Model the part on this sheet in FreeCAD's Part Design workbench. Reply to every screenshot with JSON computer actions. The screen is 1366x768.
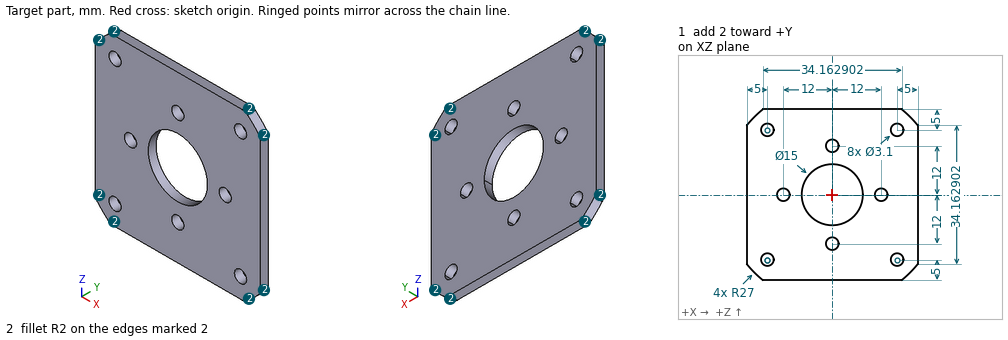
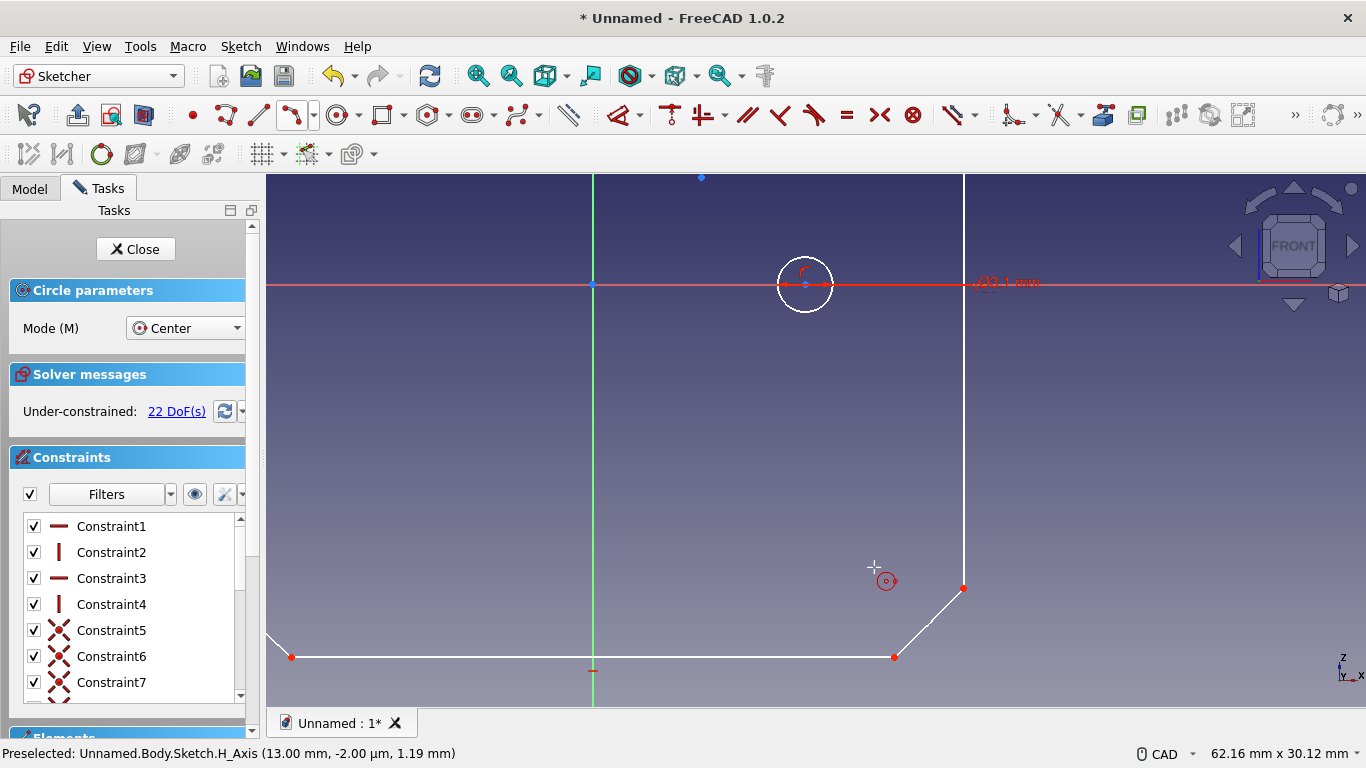
{"action": "left_click", "coordinate": [874, 566]}
{"action": "mouse_move", "coordinate": [894, 547]}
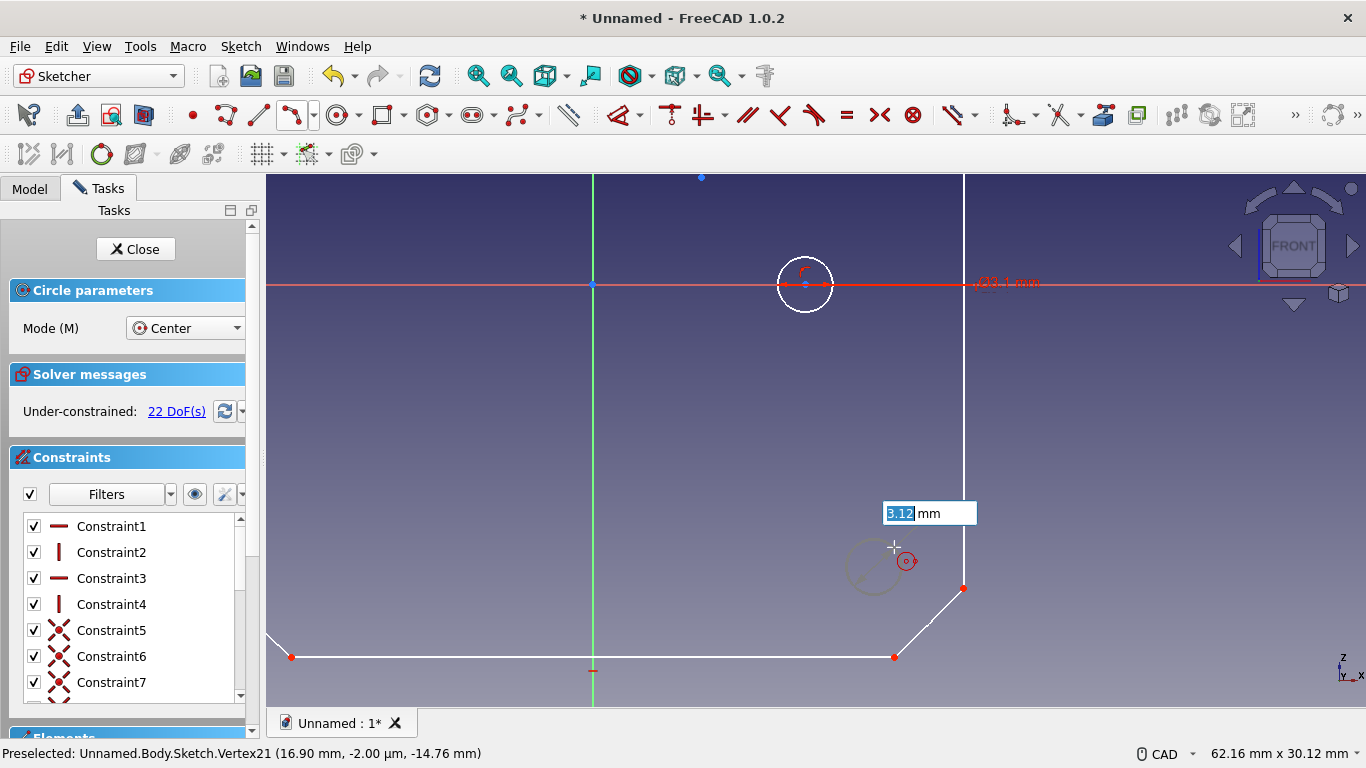
{"action": "type", "text": "3.1"}
{"action": "key", "text": "Return"}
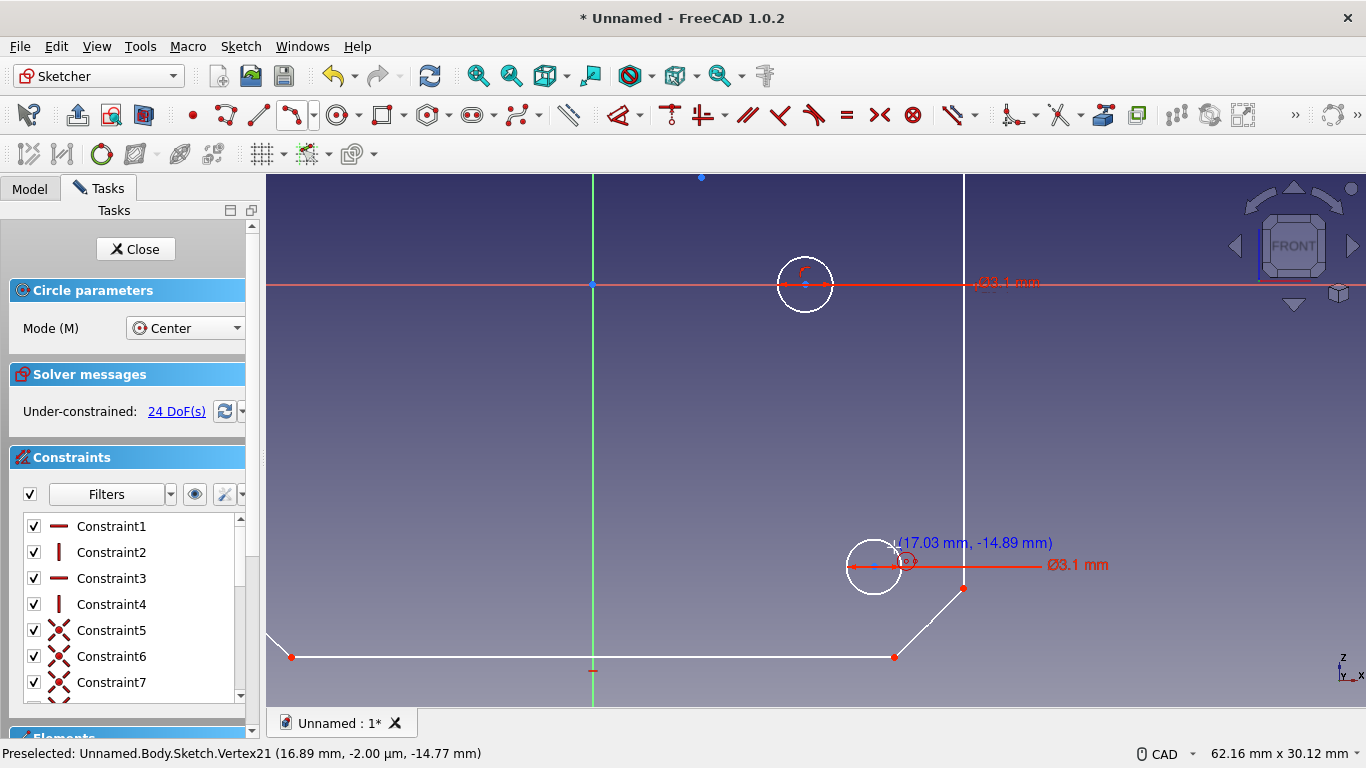
{"action": "left_click", "coordinate": [593, 285]}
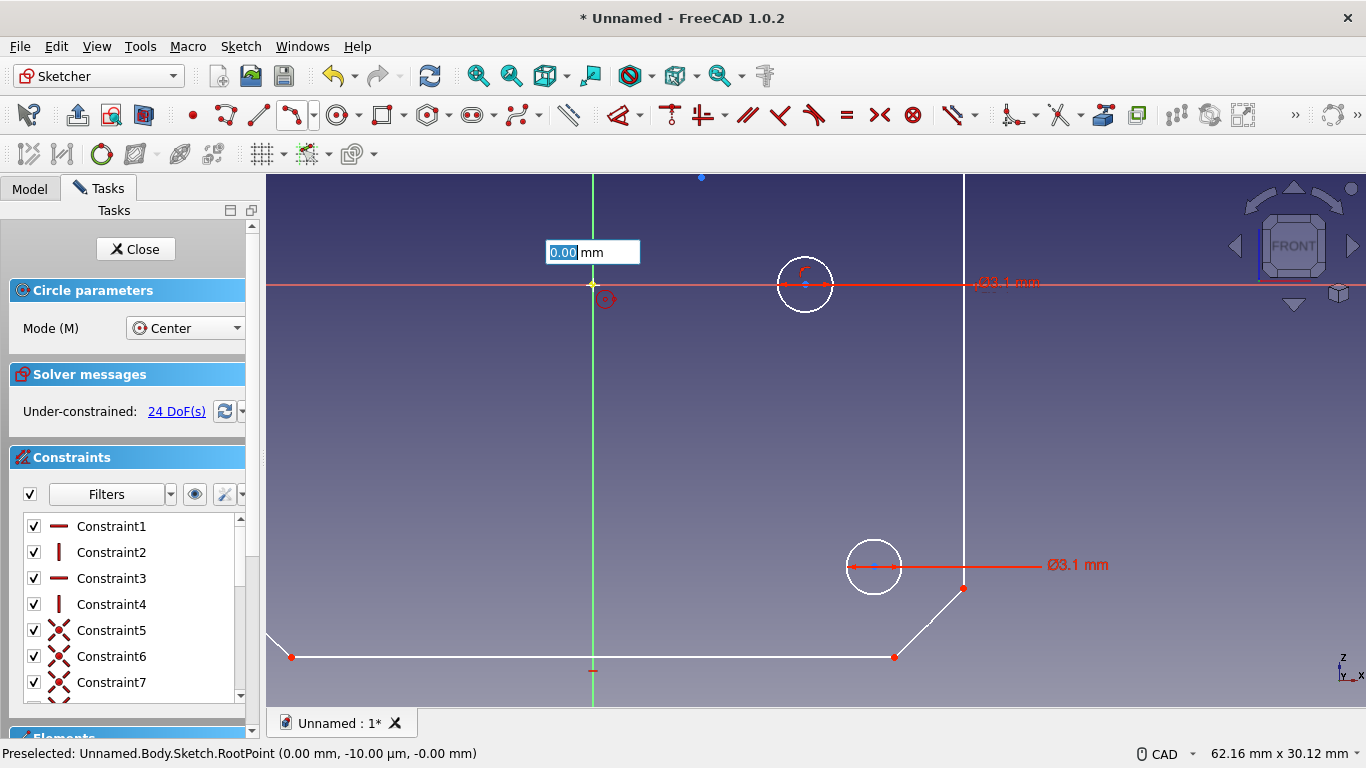
{"action": "scroll", "coordinate": [874, 568], "scroll_direction": "down", "scroll_amount": 4}
{"action": "mouse_move", "coordinate": [790, 399]}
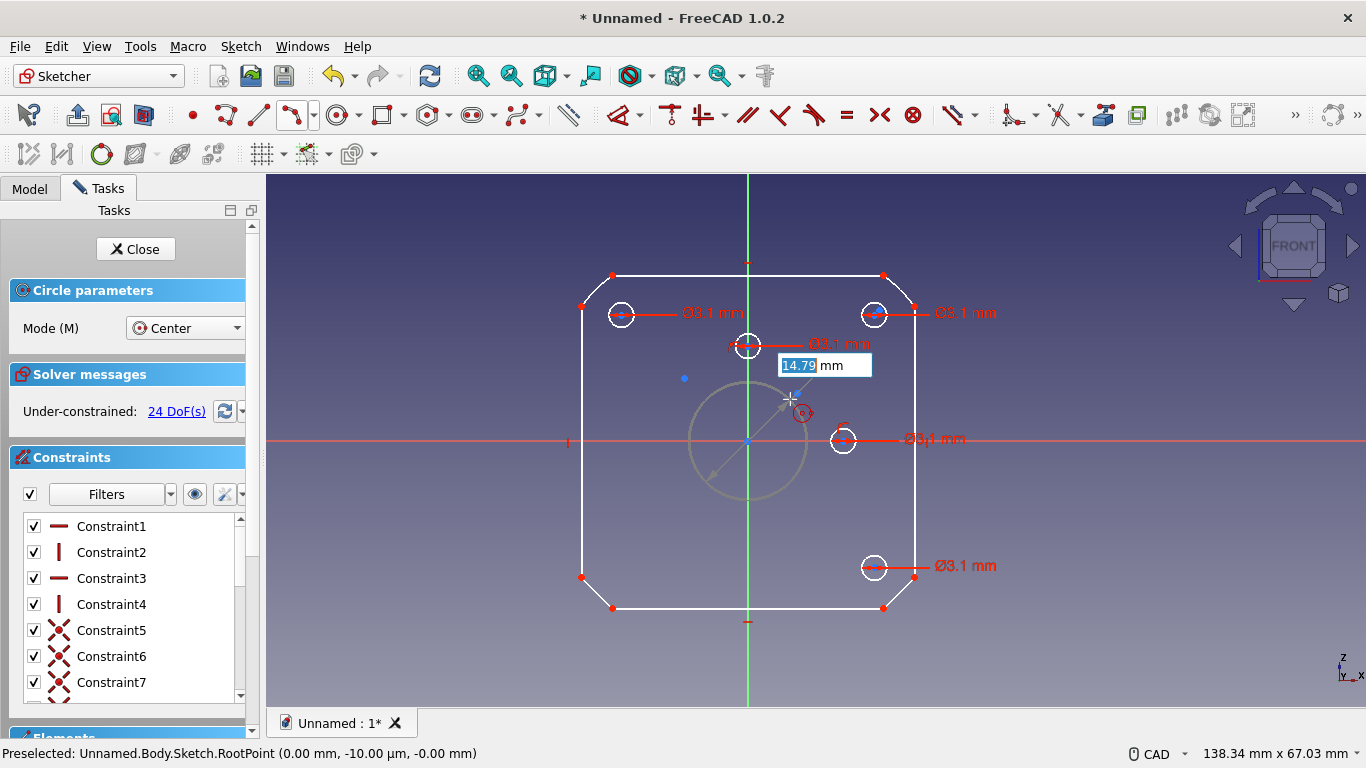
{"action": "type", "text": "15"}
{"action": "key", "text": "Return"}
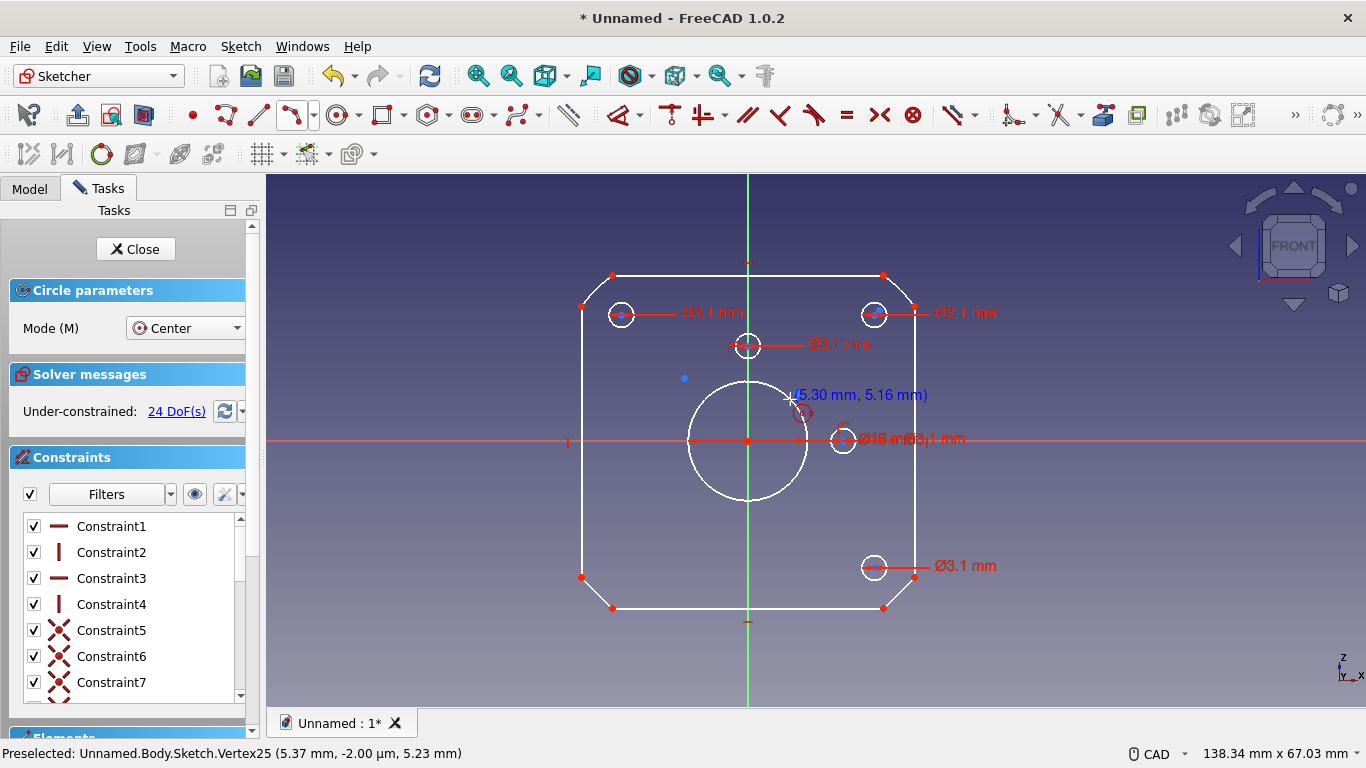
{"action": "scroll", "coordinate": [652, 441], "scroll_direction": "up", "scroll_amount": 4}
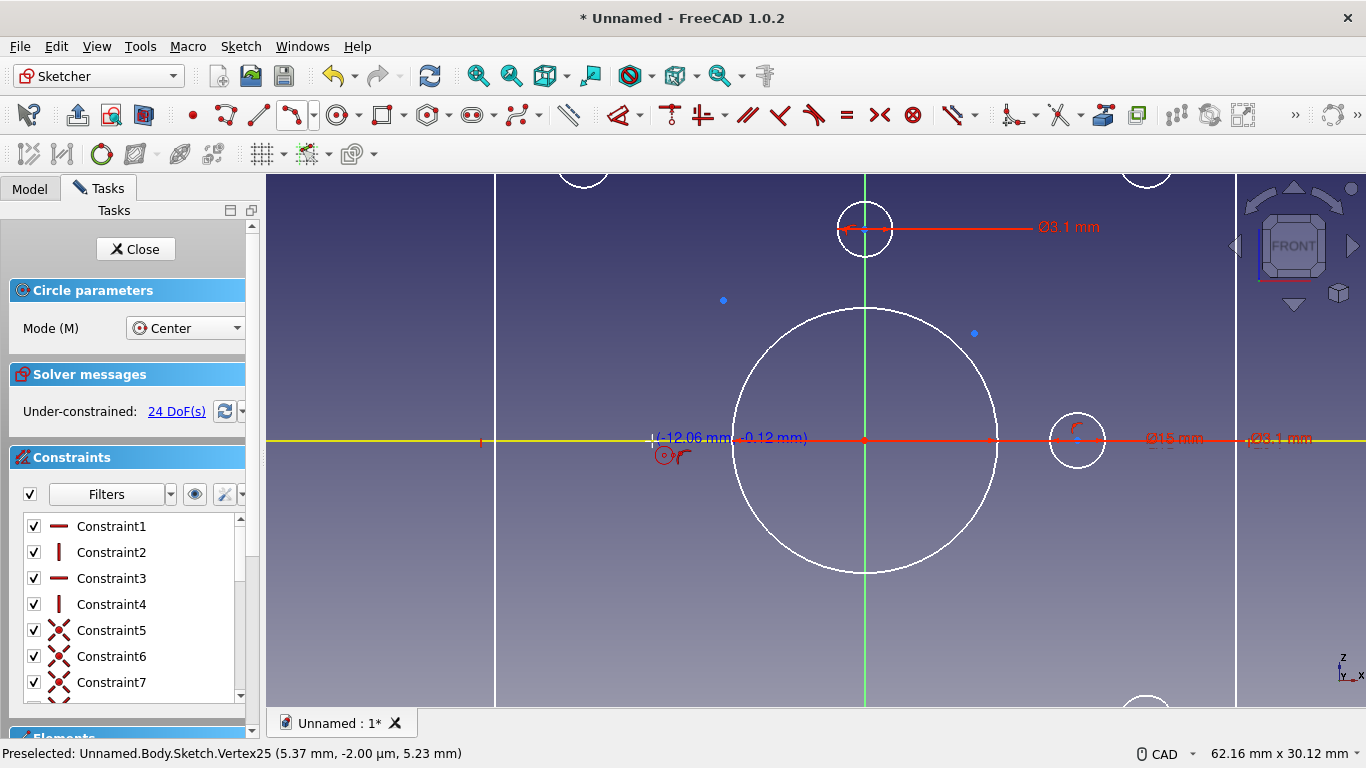
{"action": "left_click", "coordinate": [653, 441]}
{"action": "mouse_move", "coordinate": [672, 421]}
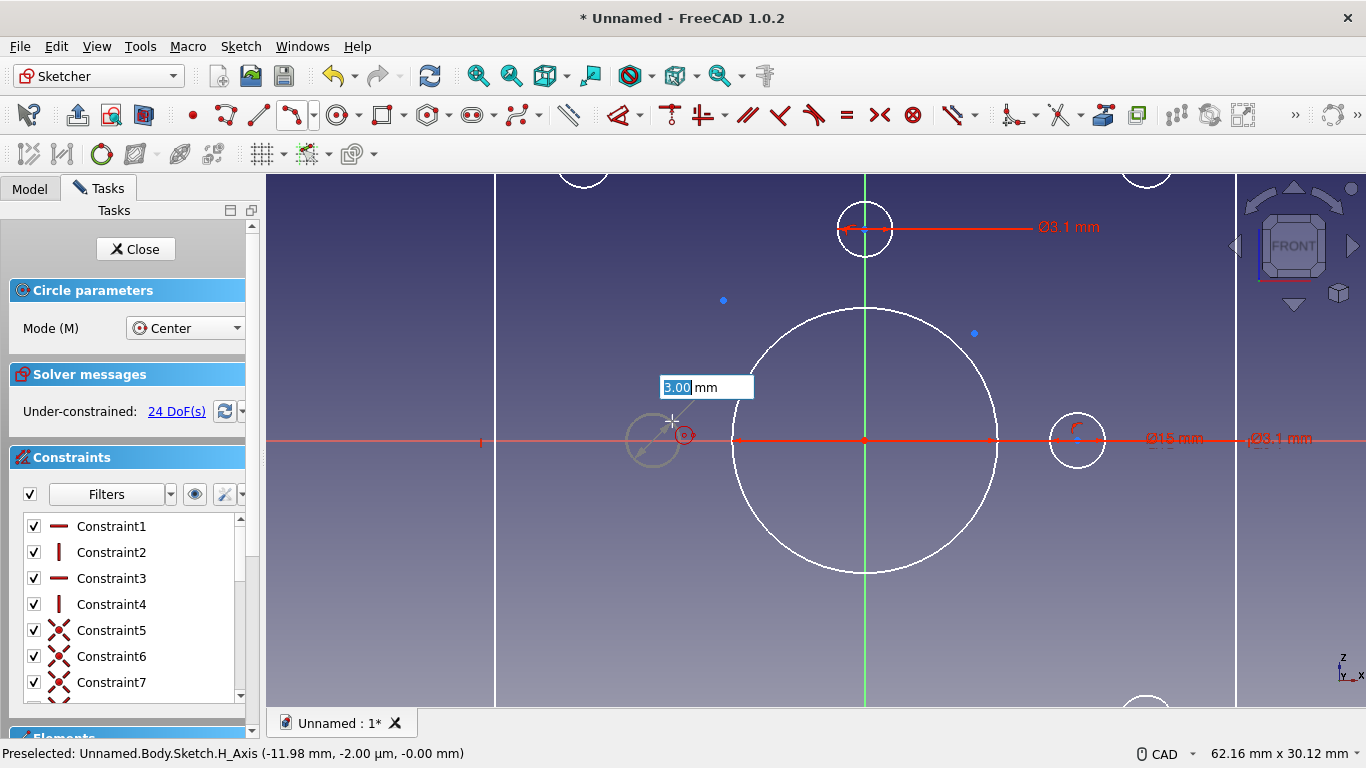
{"action": "type", "text": "3.1"}
{"action": "key", "text": "Return"}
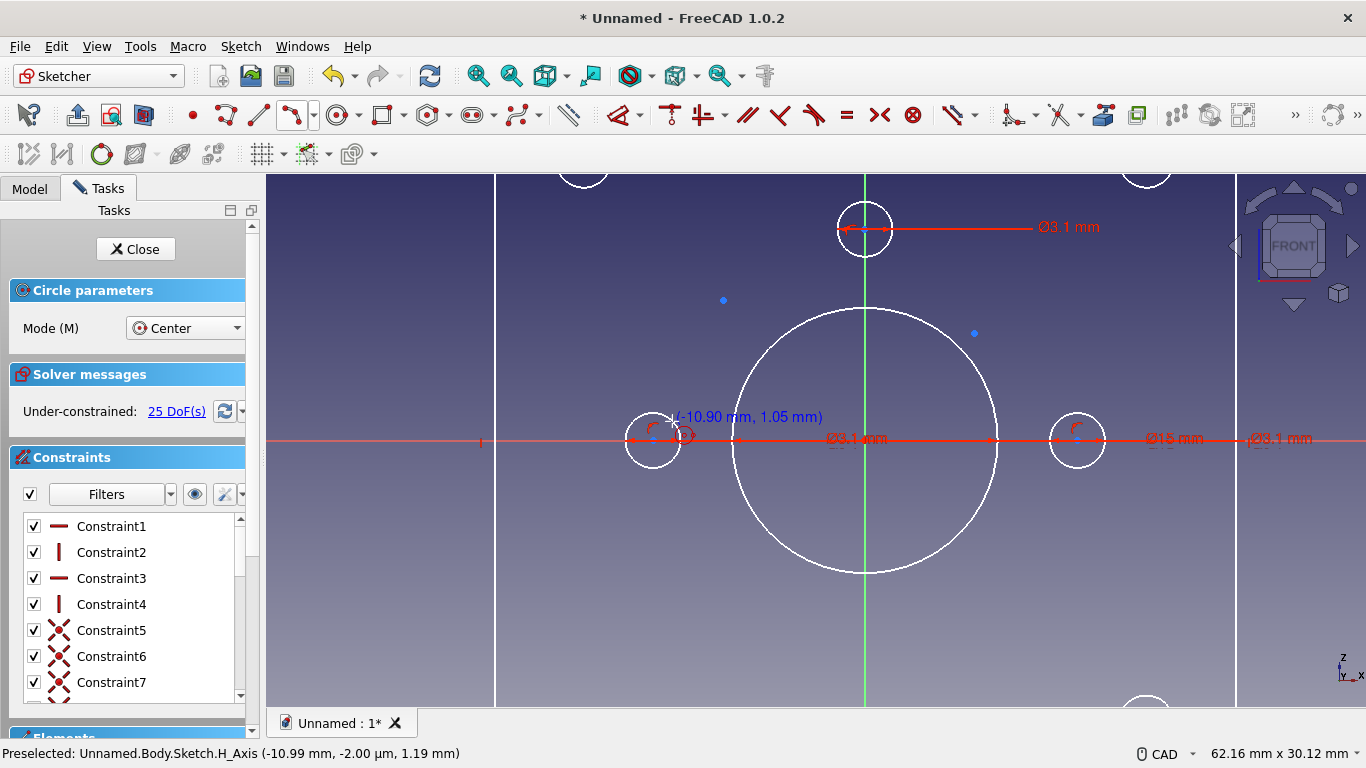
{"action": "left_click", "coordinate": [865, 653]}
{"action": "mouse_move", "coordinate": [884, 633]}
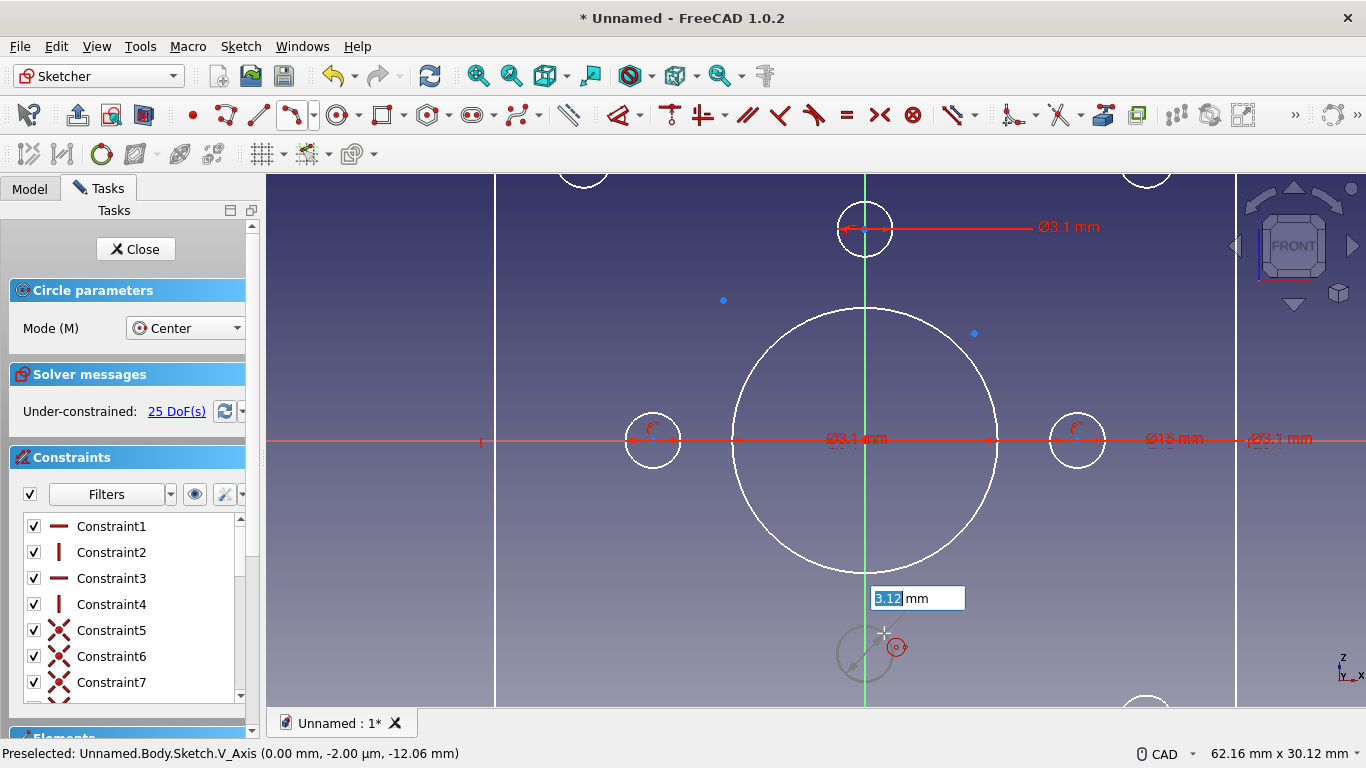
{"action": "type", "text": "3.1"}
{"action": "key", "text": "Return"}